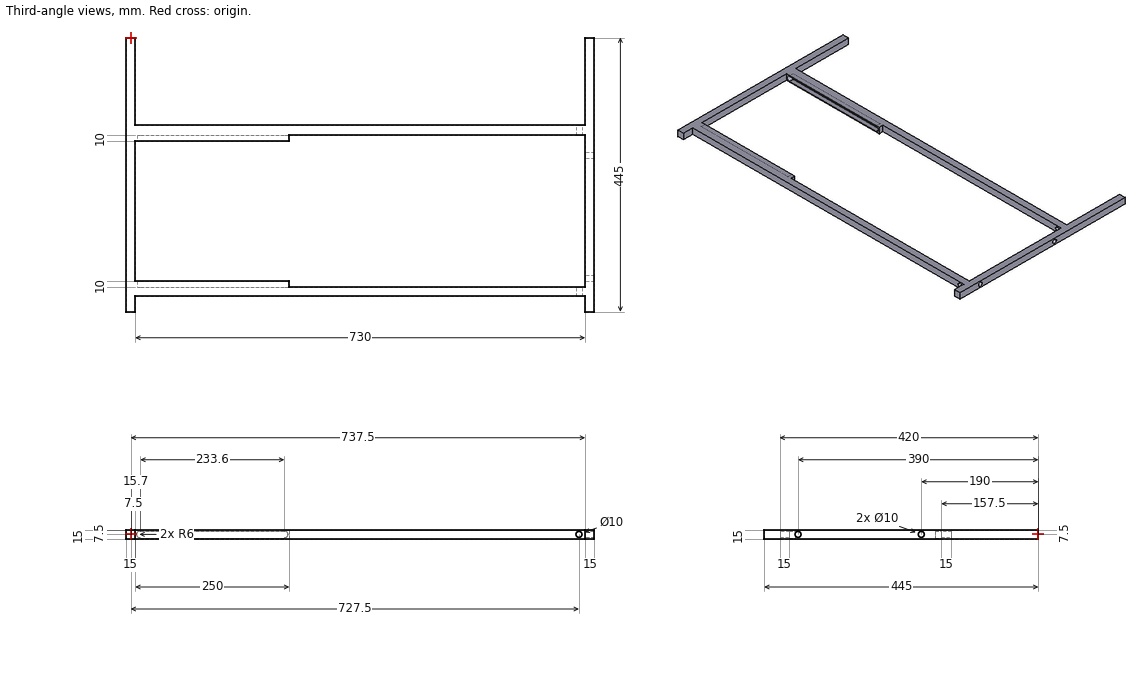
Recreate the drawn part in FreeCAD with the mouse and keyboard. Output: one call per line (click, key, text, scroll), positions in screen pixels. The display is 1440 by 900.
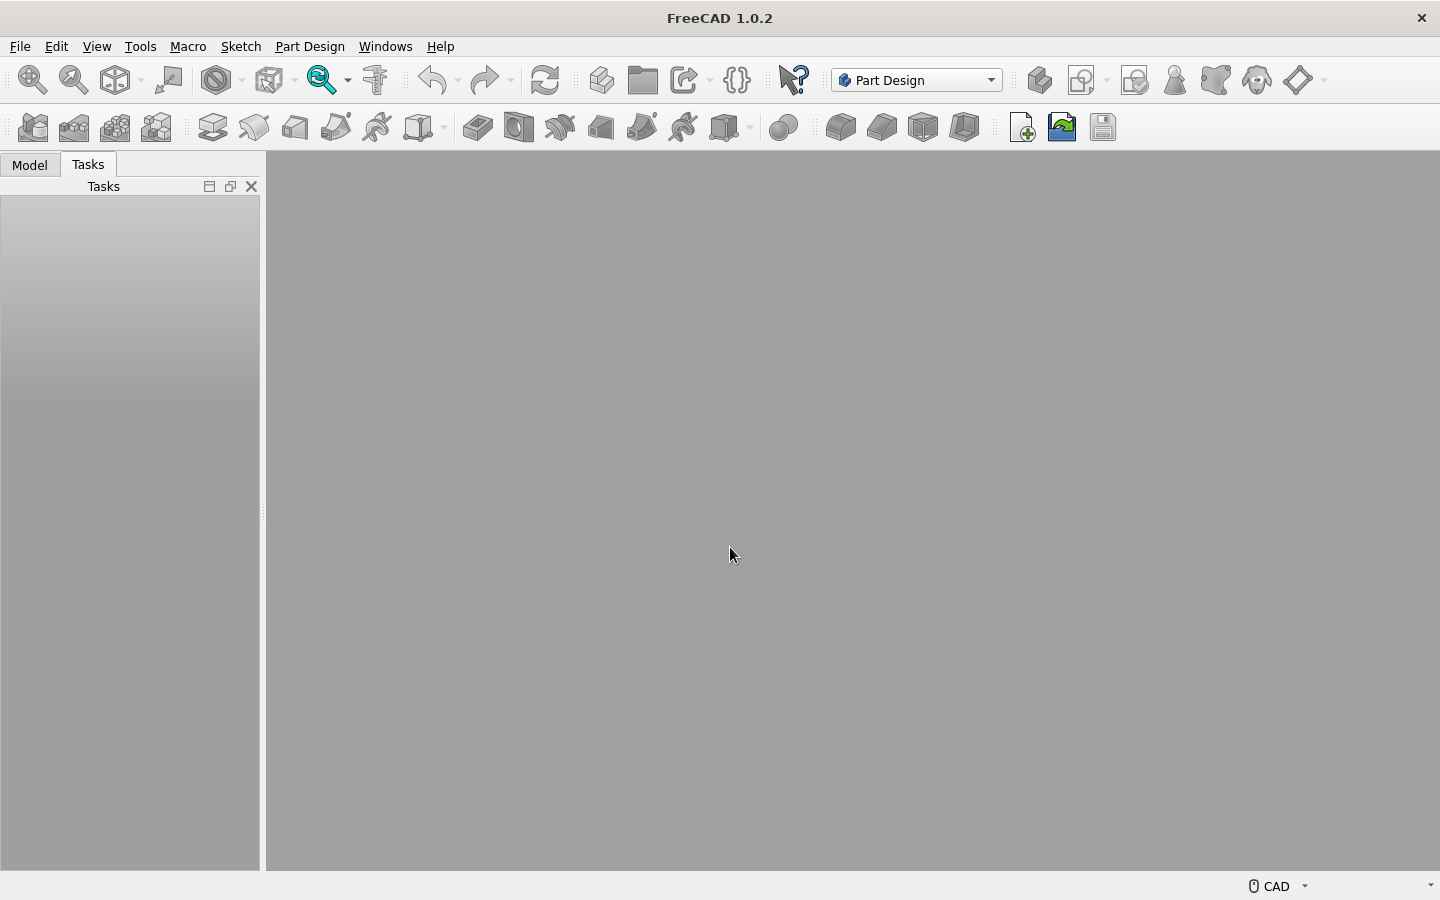
click(1021, 128)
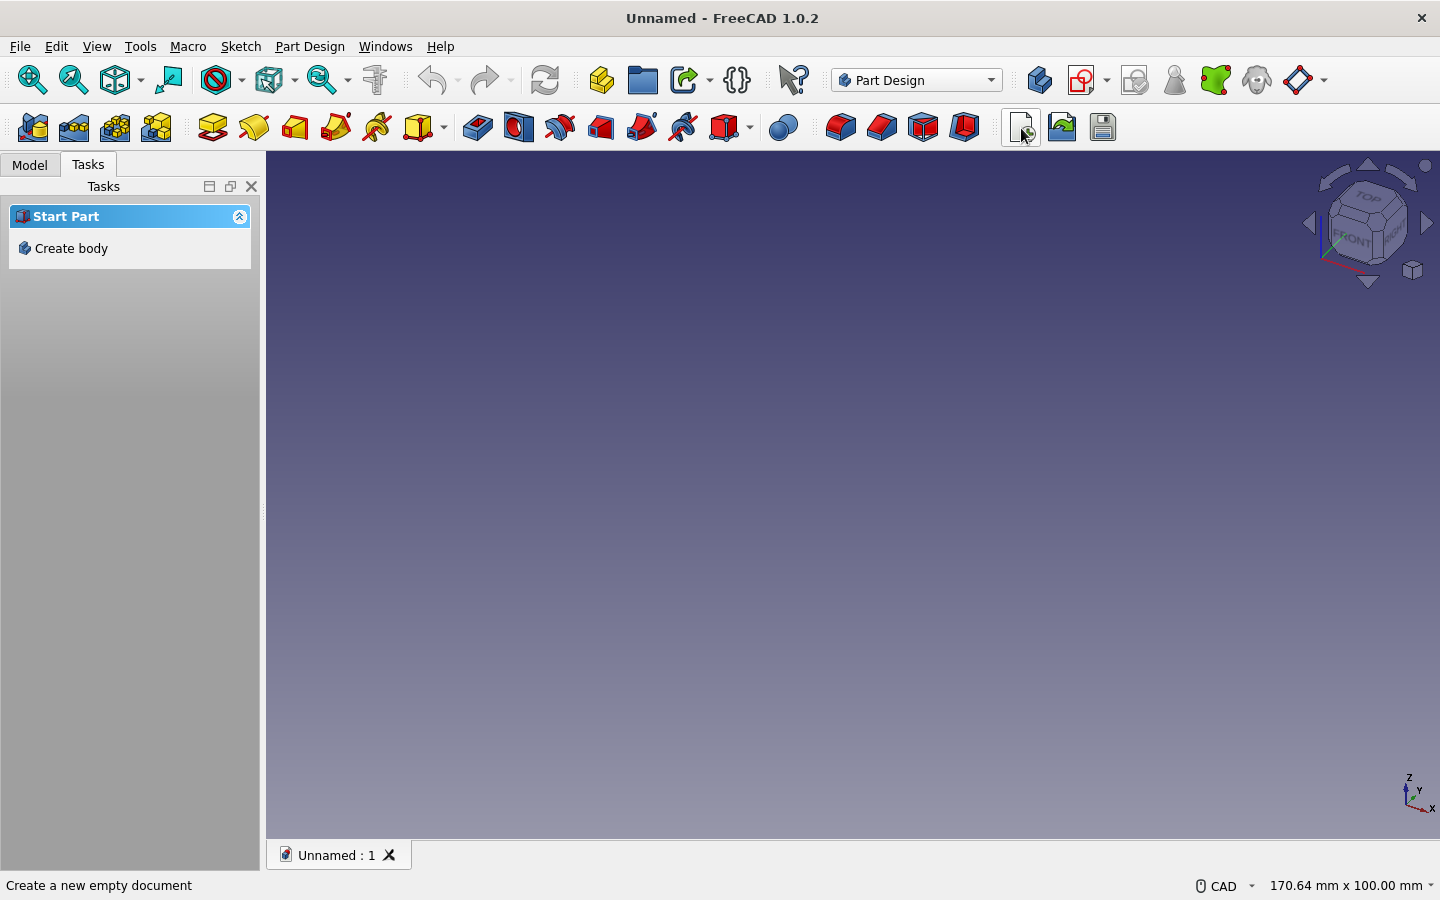
click(1080, 80)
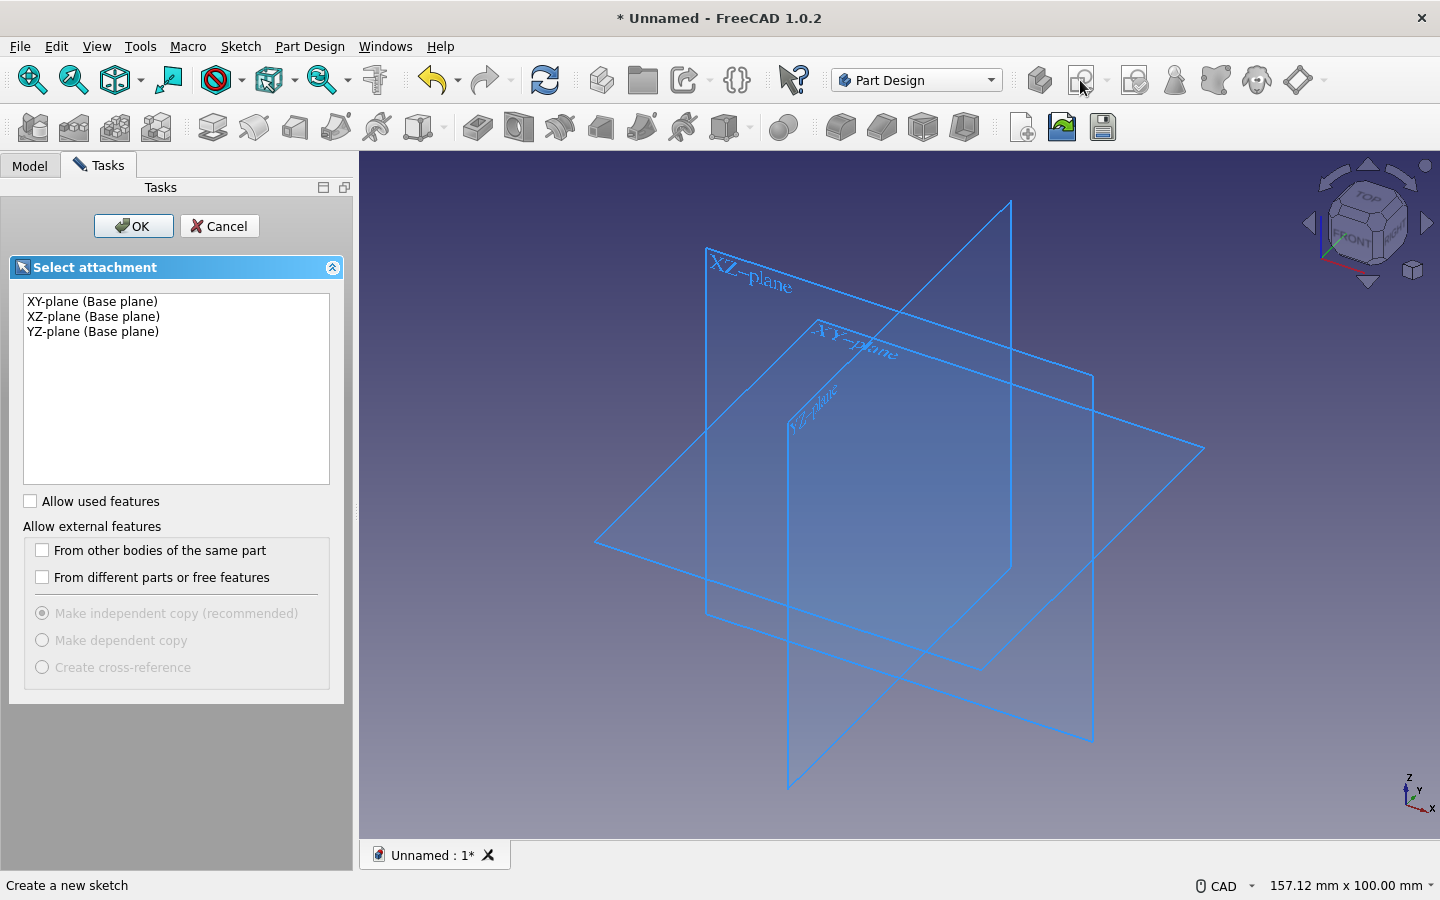
click(84, 316)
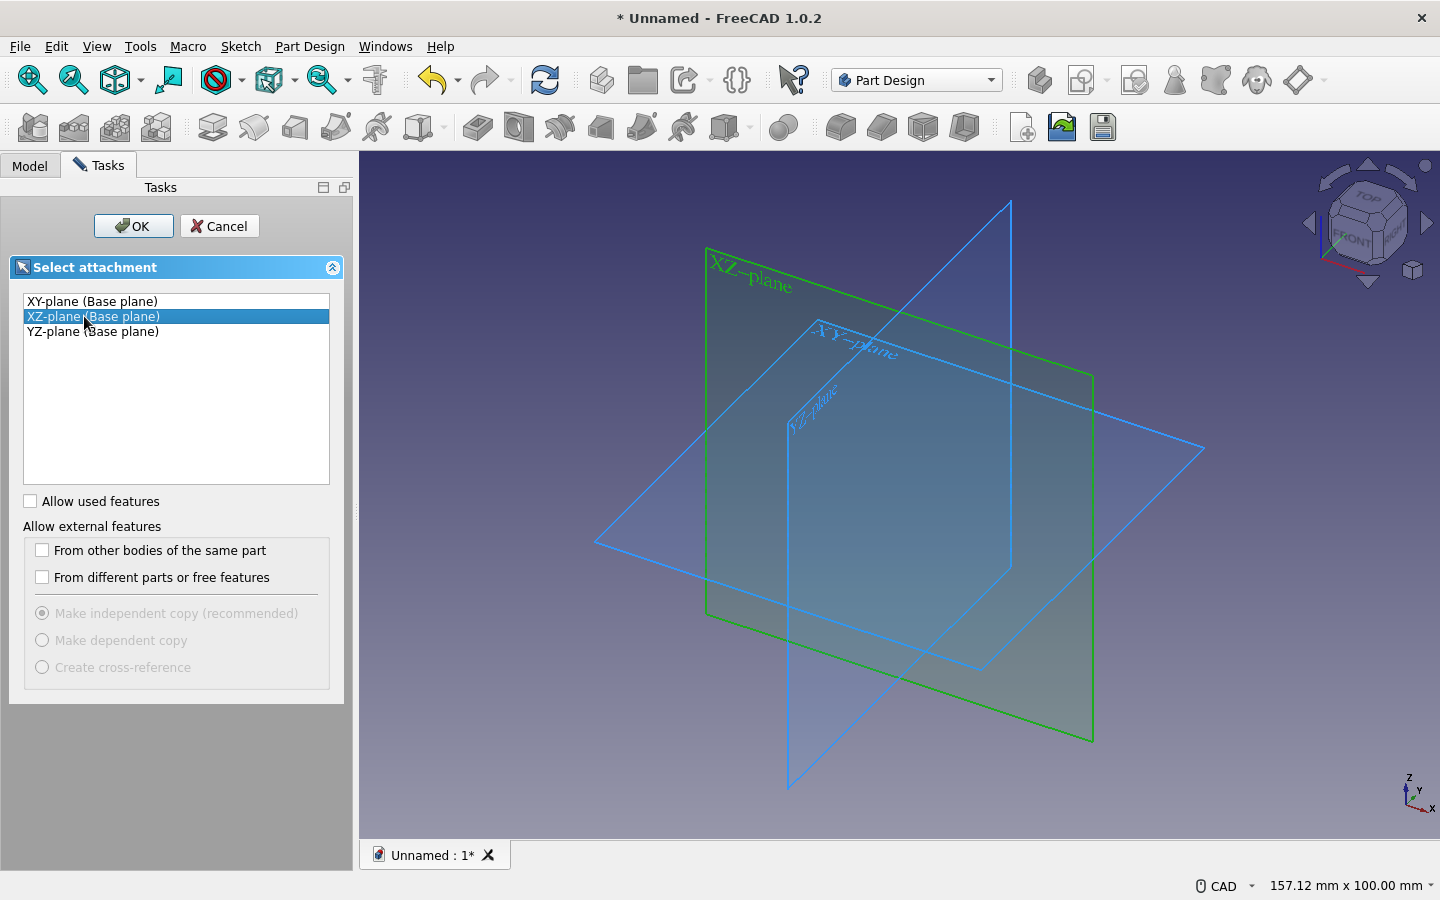
click(134, 226)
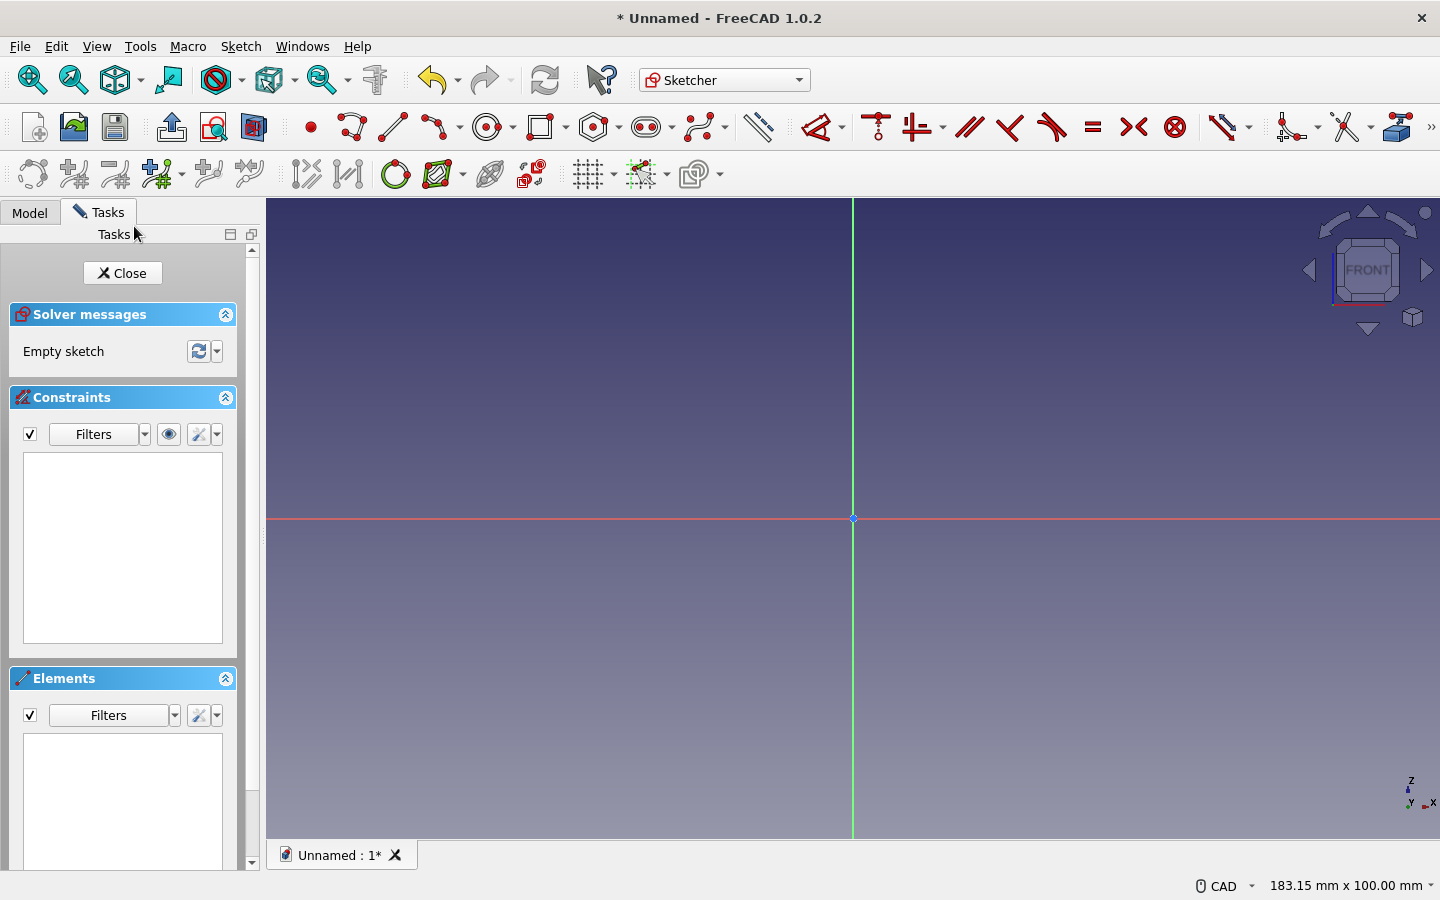
scroll(875, 518, up, 7)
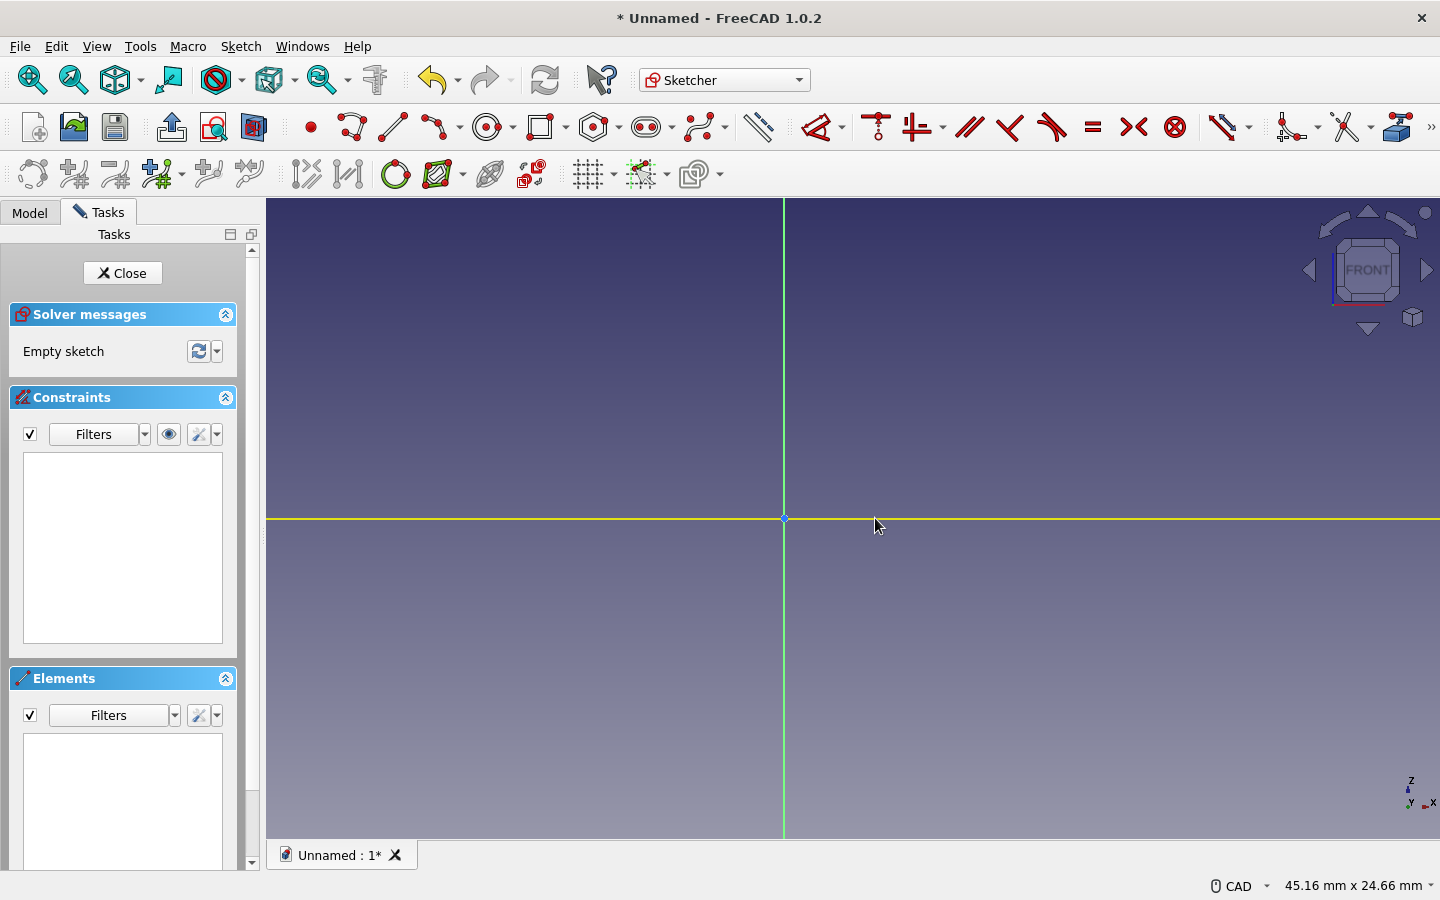
click(566, 128)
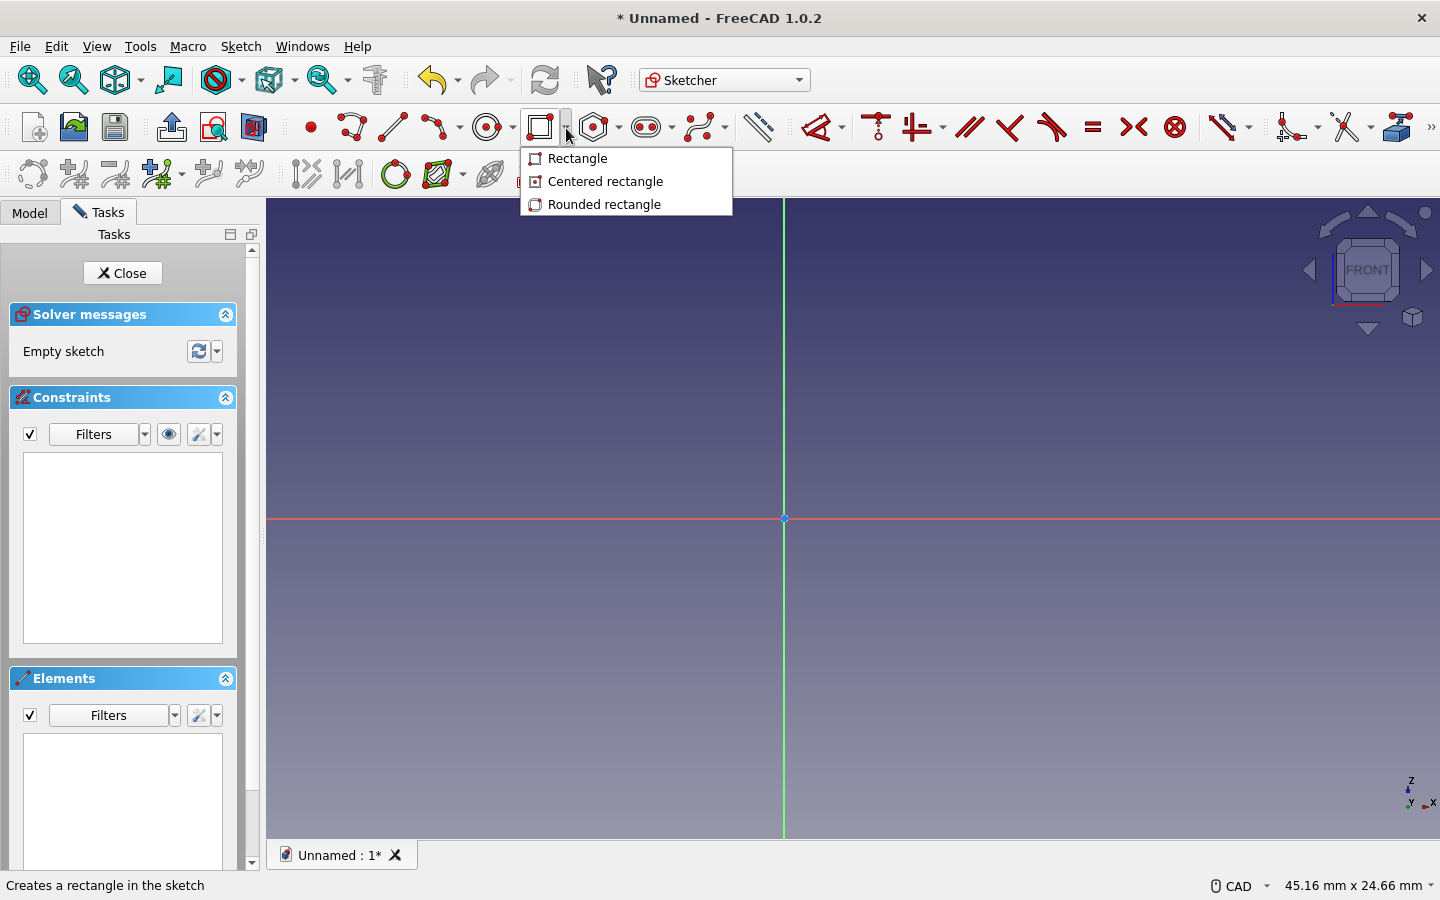
click(626, 182)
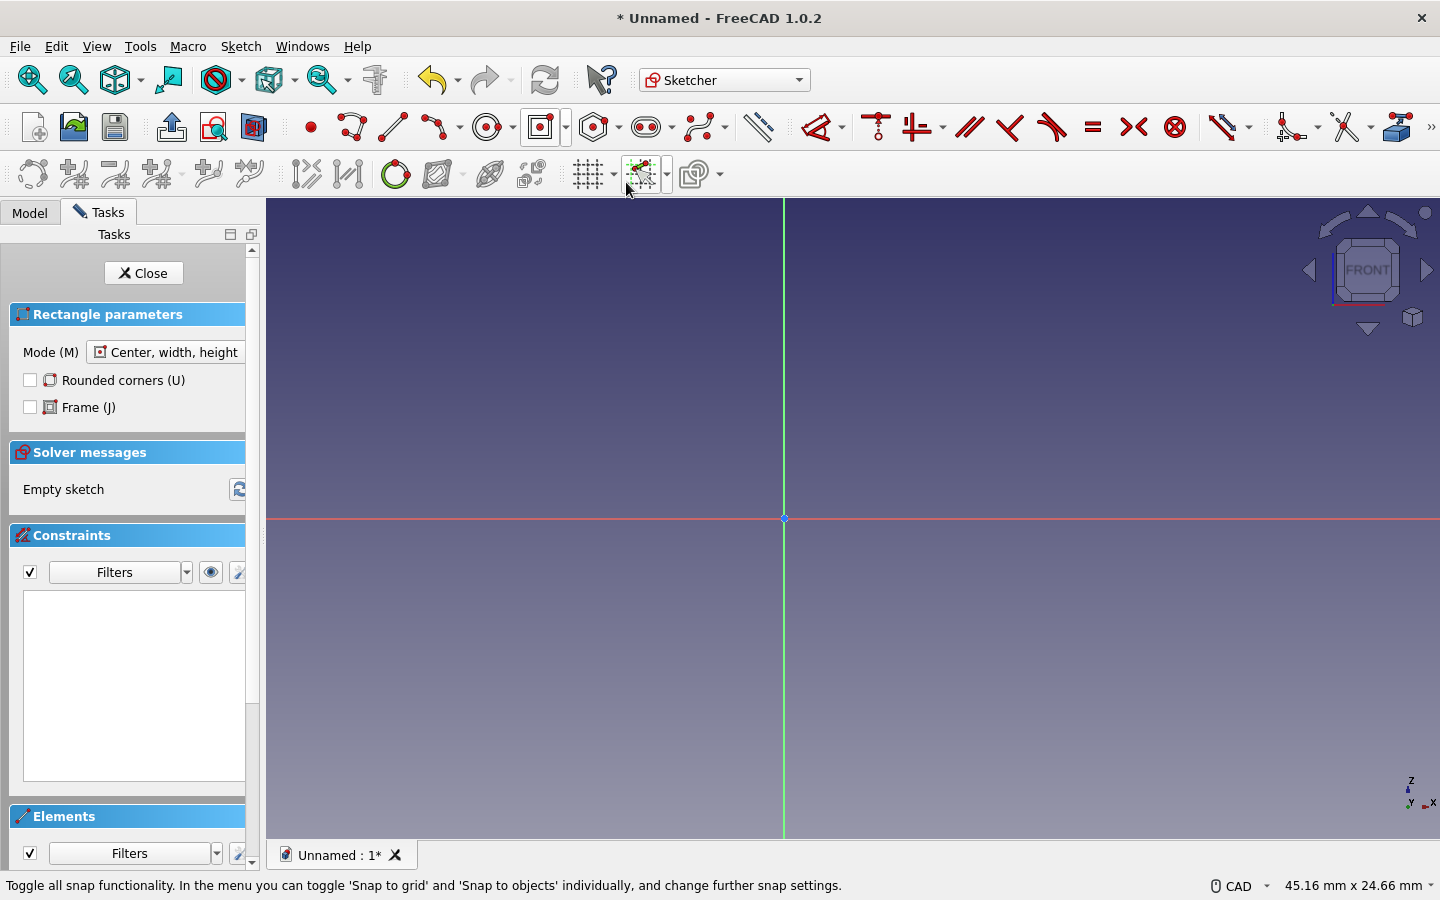
click(784, 518)
click(979, 324)
key(Escape)